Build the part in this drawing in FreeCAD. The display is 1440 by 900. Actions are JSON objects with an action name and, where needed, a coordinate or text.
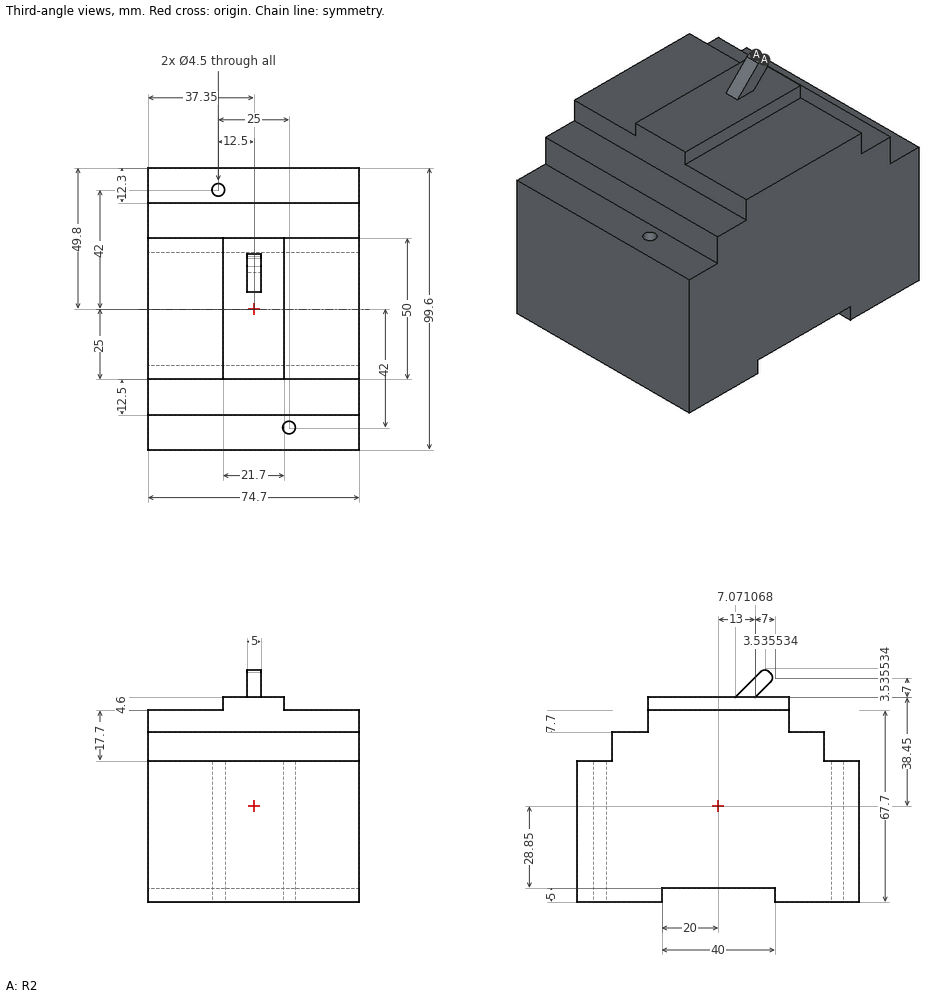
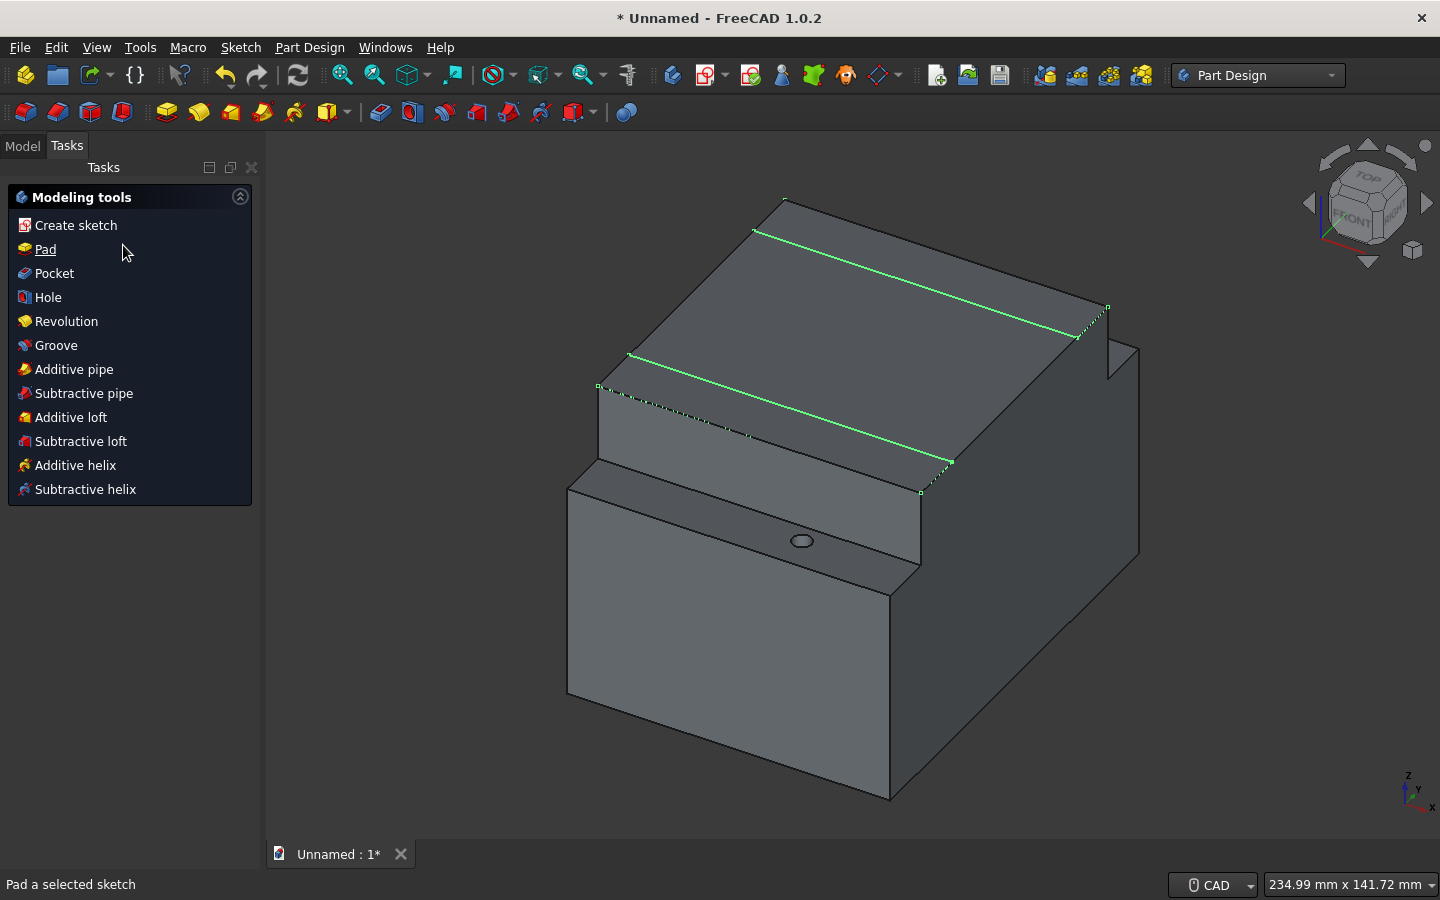
{"action": "left_click", "coordinate": [382, 112]}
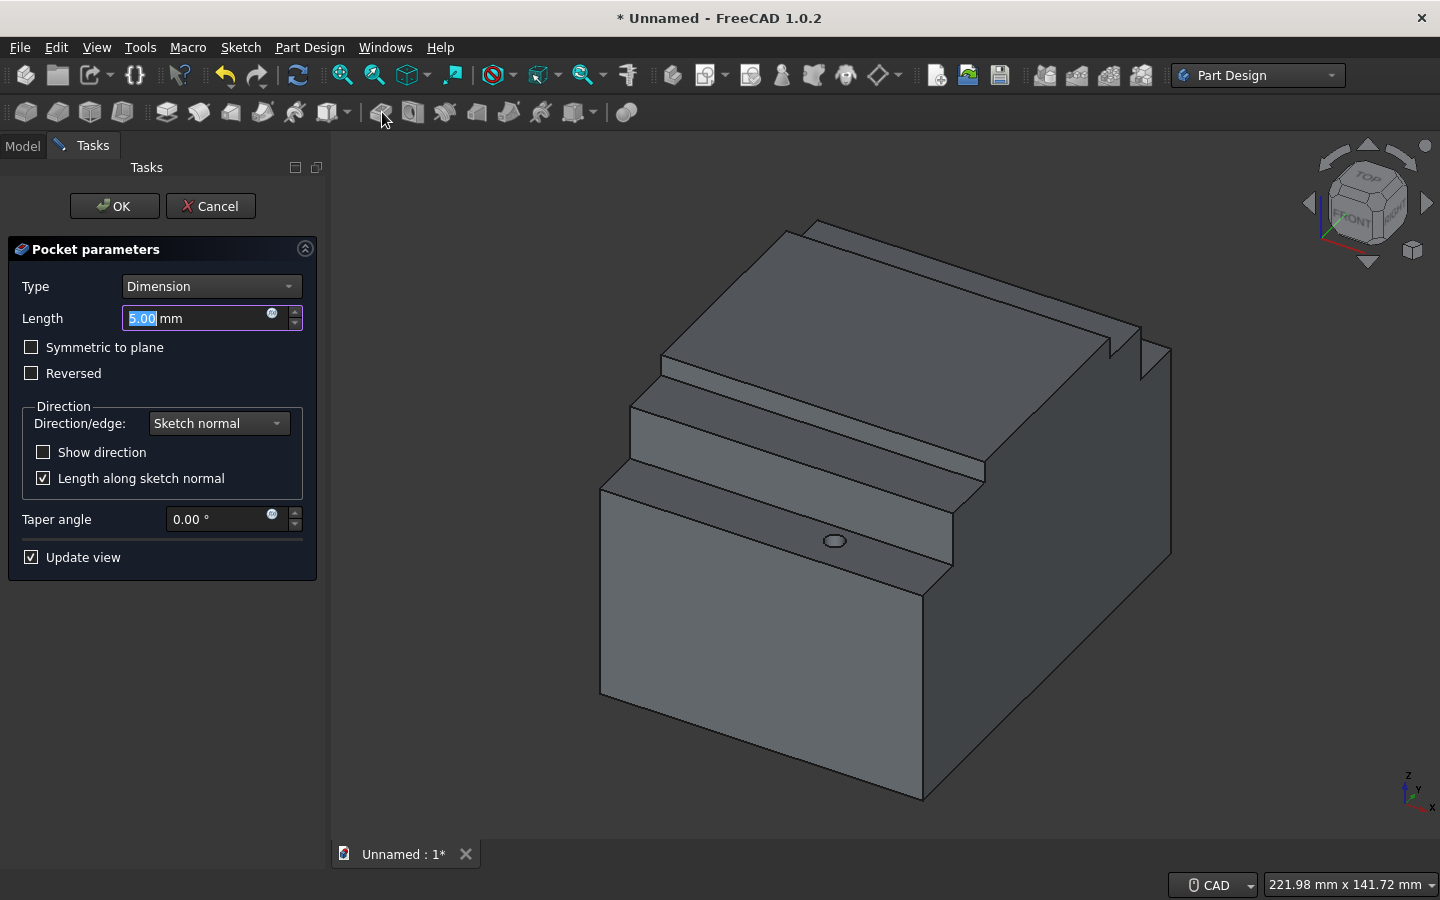
{"action": "type", "text": "7.7"}
{"action": "key", "text": "Tab"}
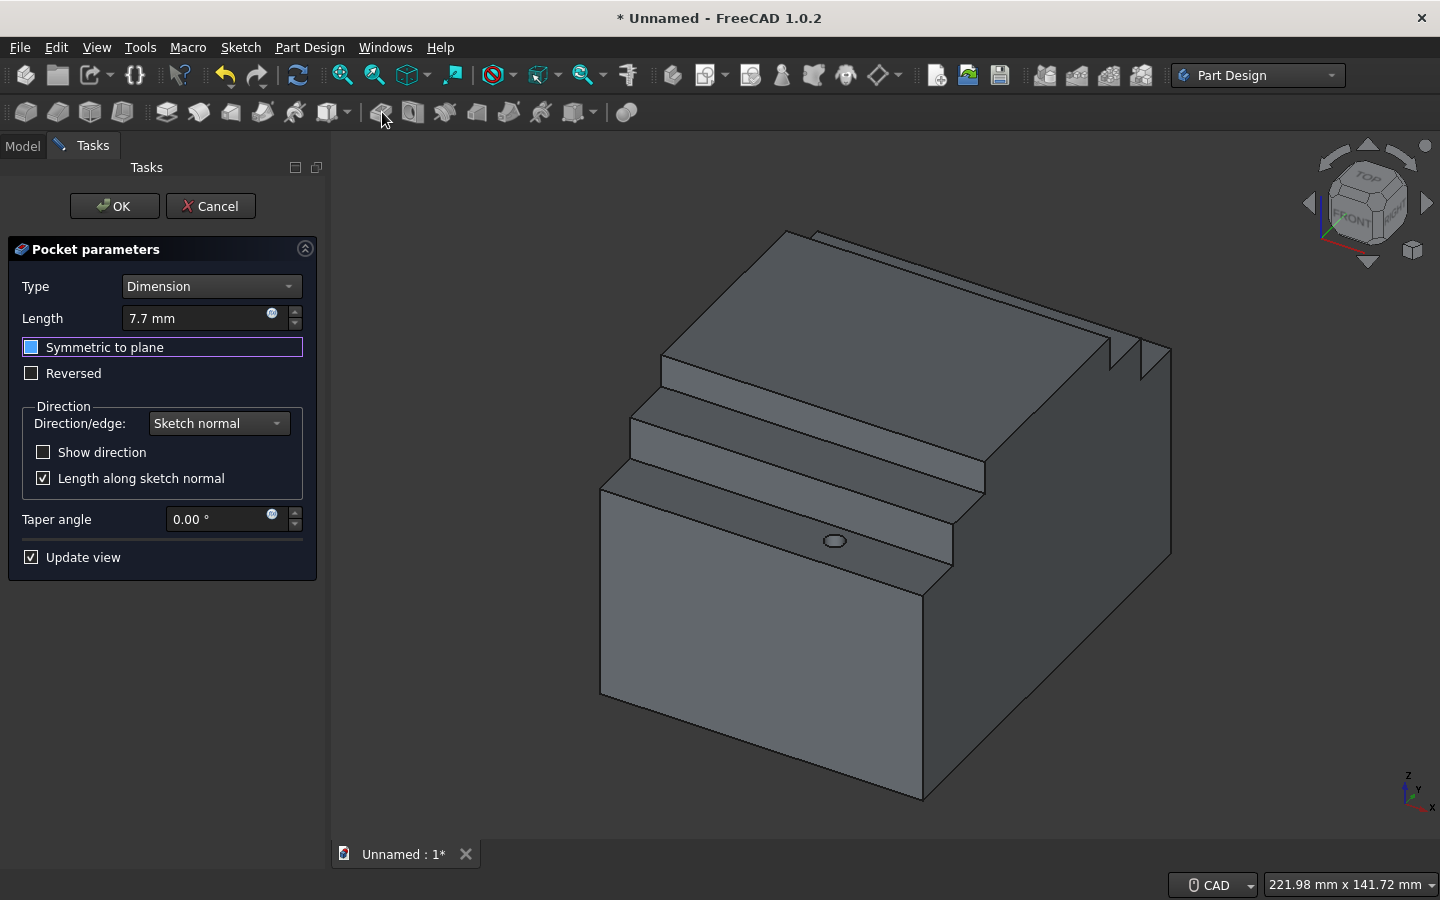
{"action": "left_click", "coordinate": [115, 206]}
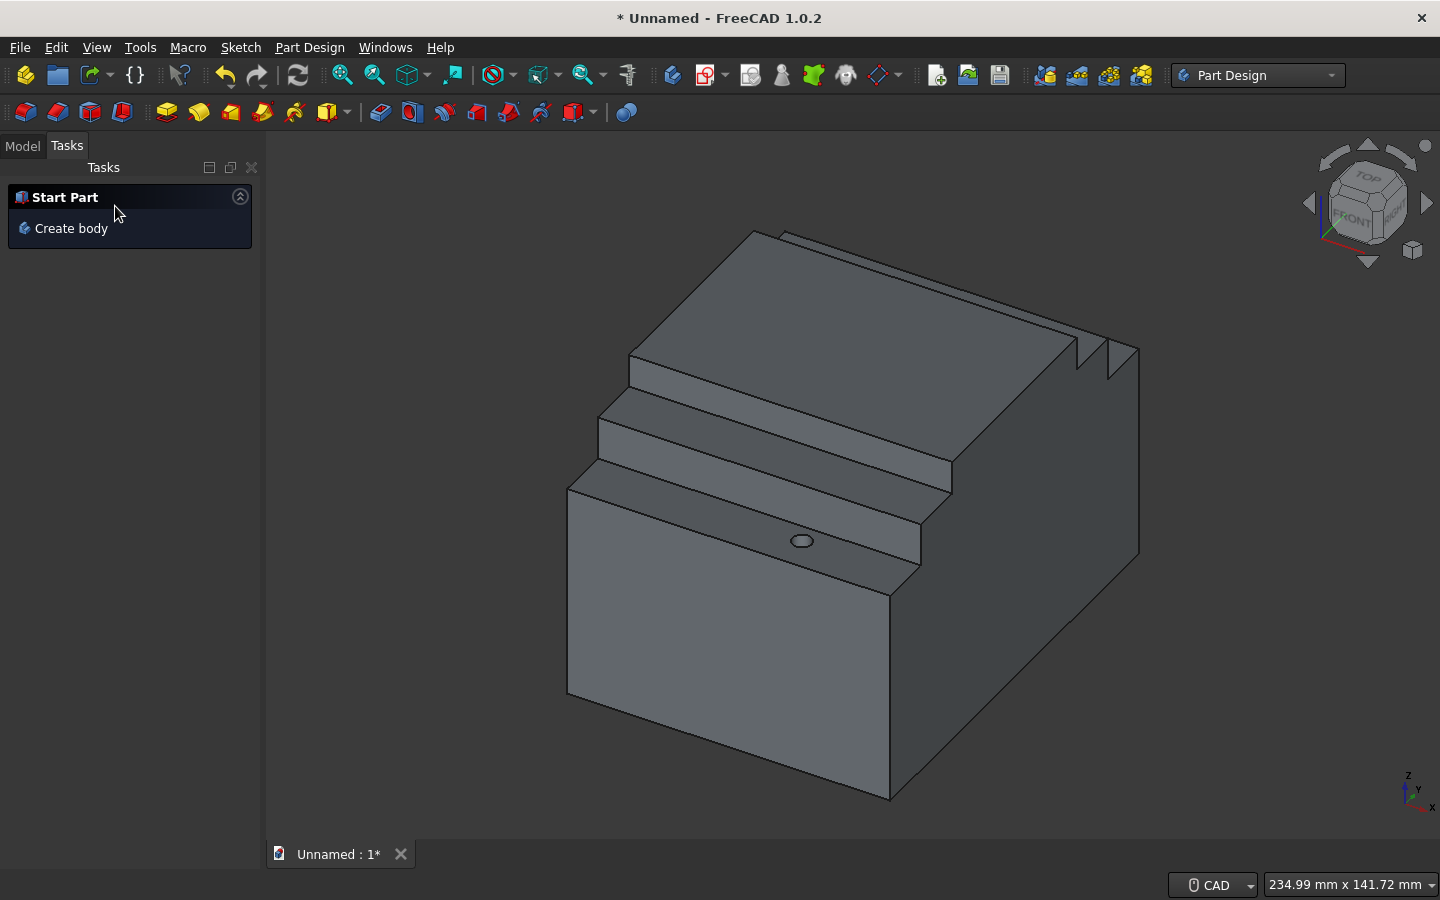
{"action": "left_click", "coordinate": [899, 361]}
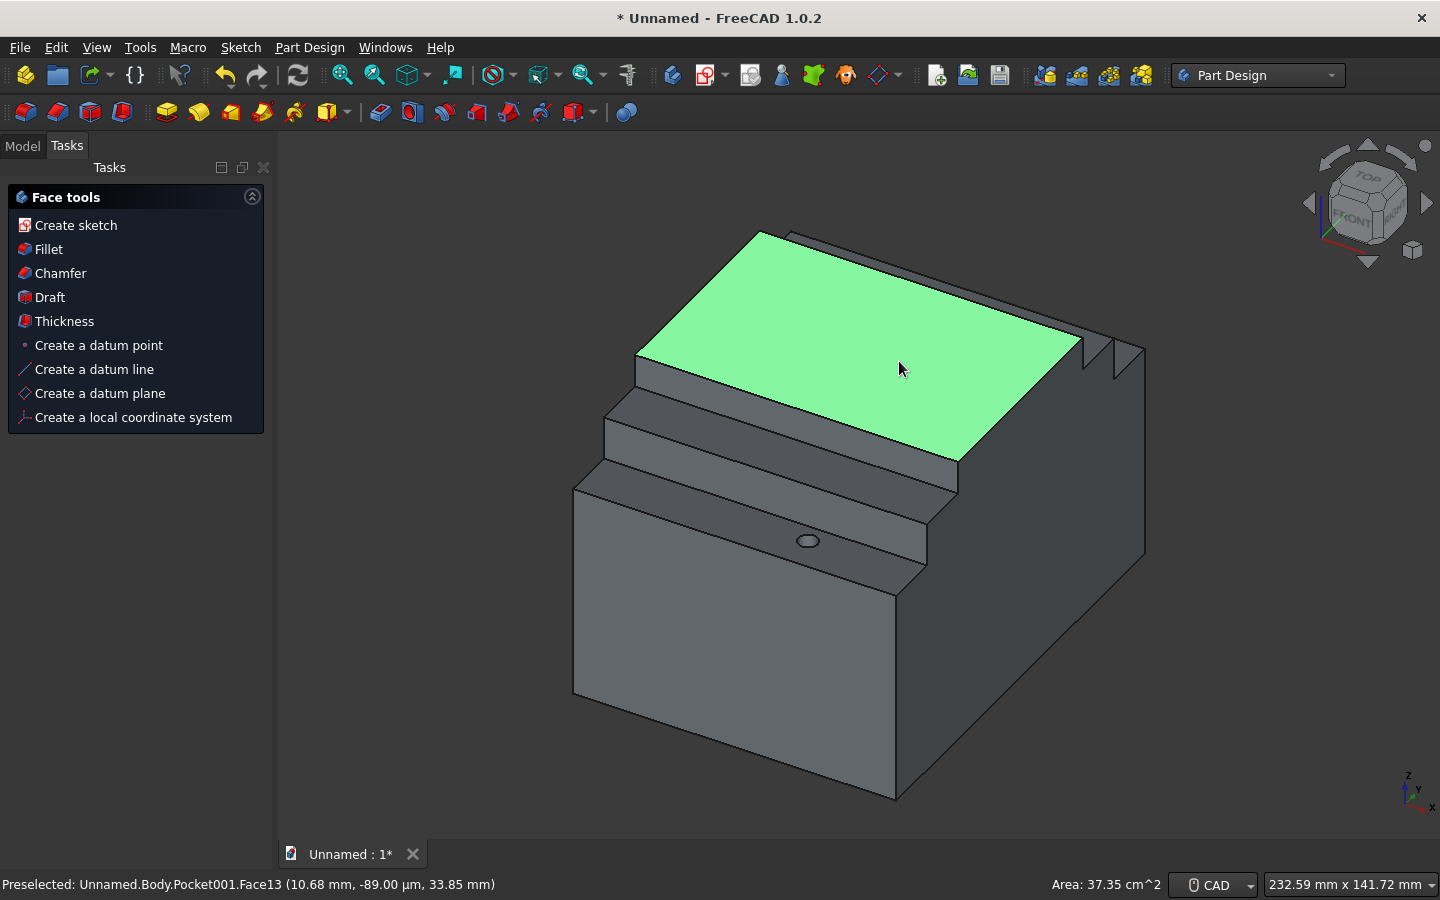
{"action": "left_click", "coordinate": [706, 76]}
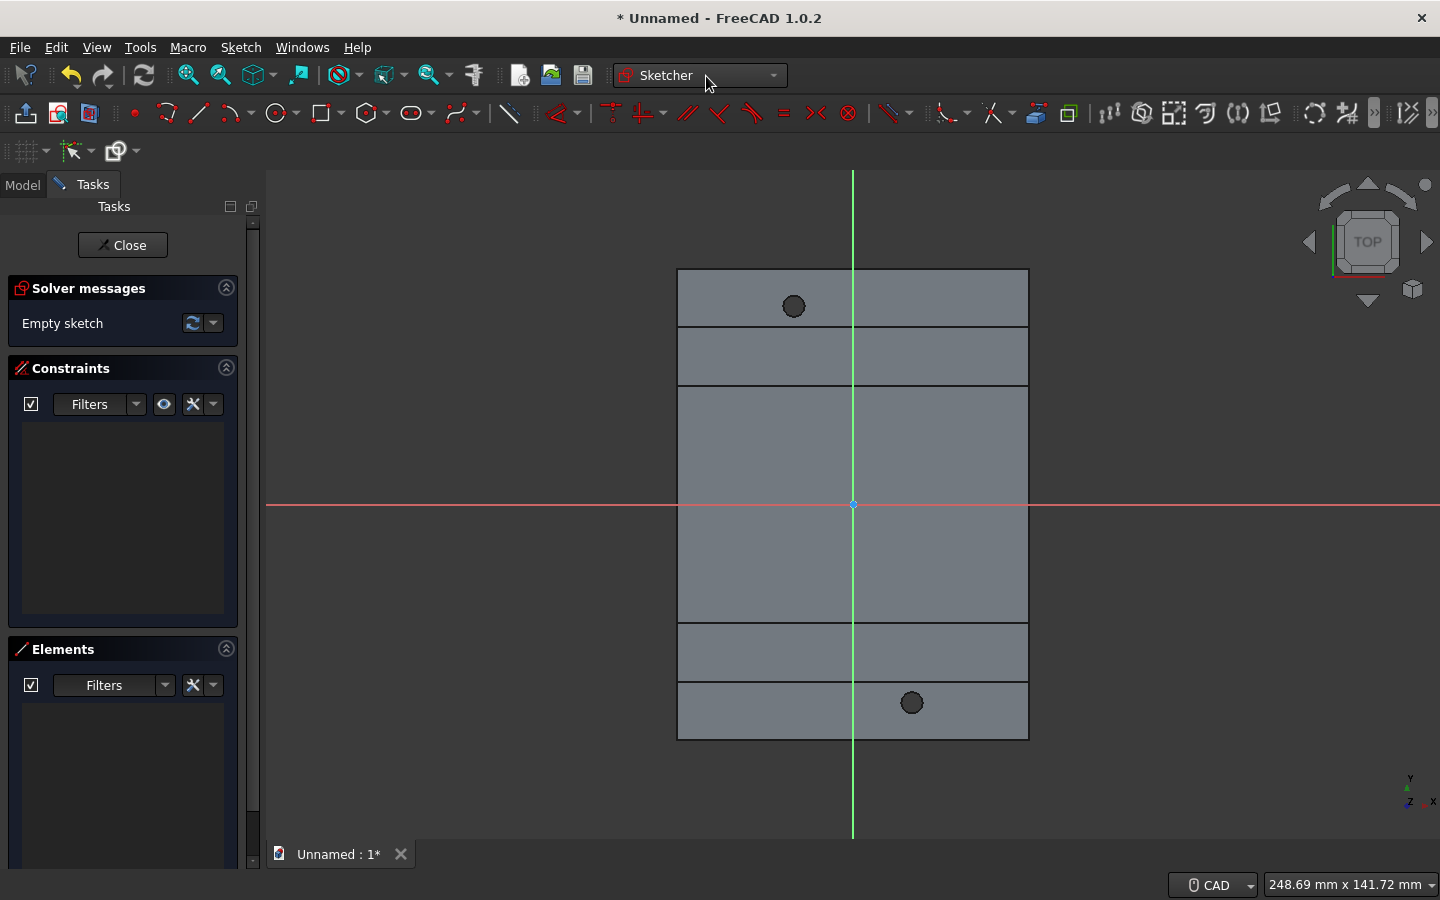
{"action": "scroll", "coordinate": [936, 505], "scroll_direction": "up", "scroll_amount": 3}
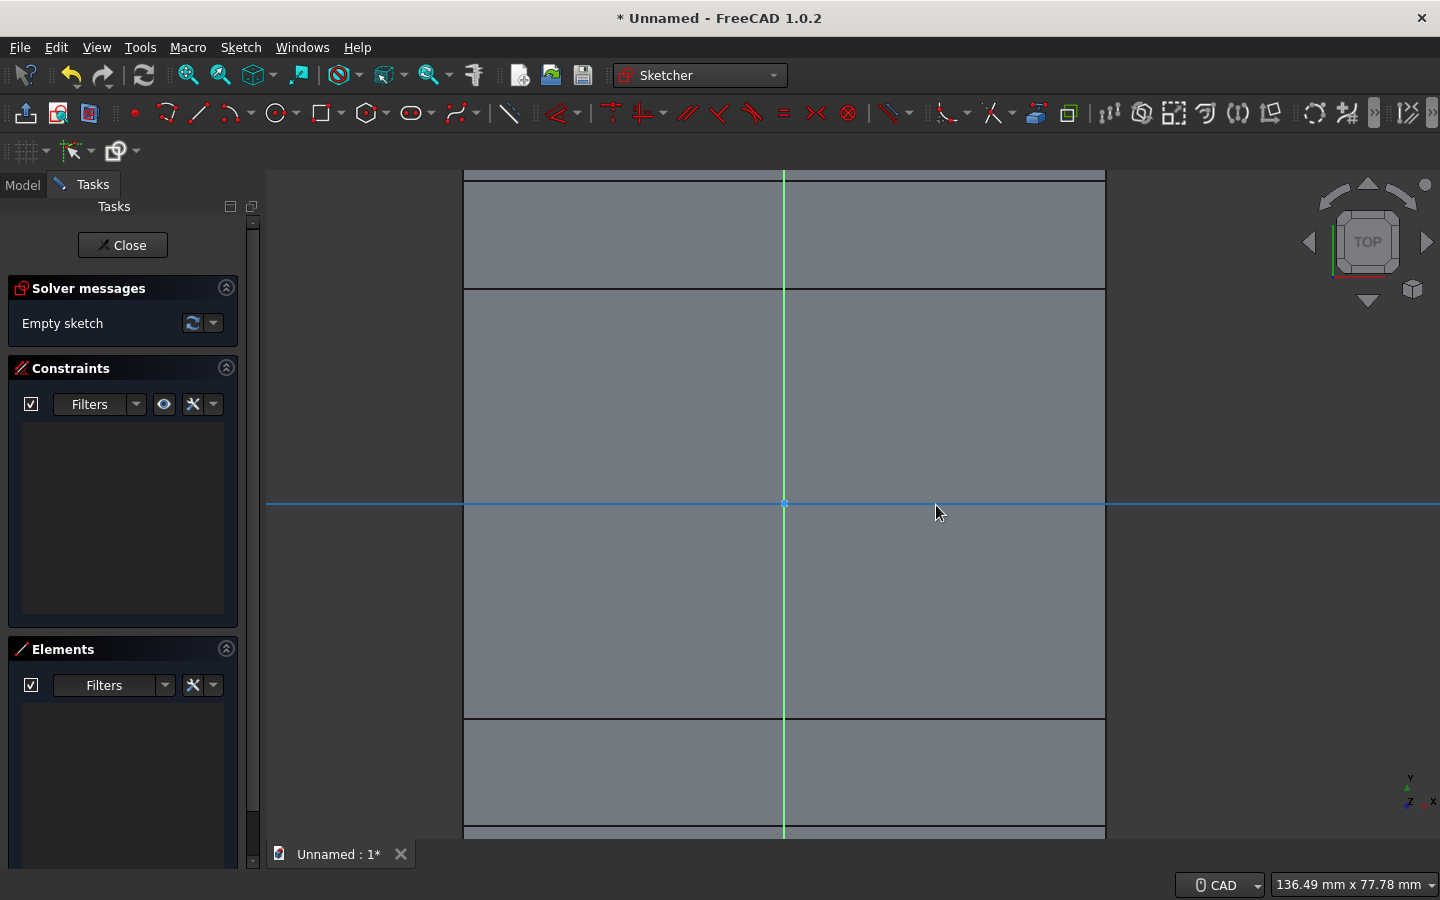
{"action": "key", "text": "g v"}